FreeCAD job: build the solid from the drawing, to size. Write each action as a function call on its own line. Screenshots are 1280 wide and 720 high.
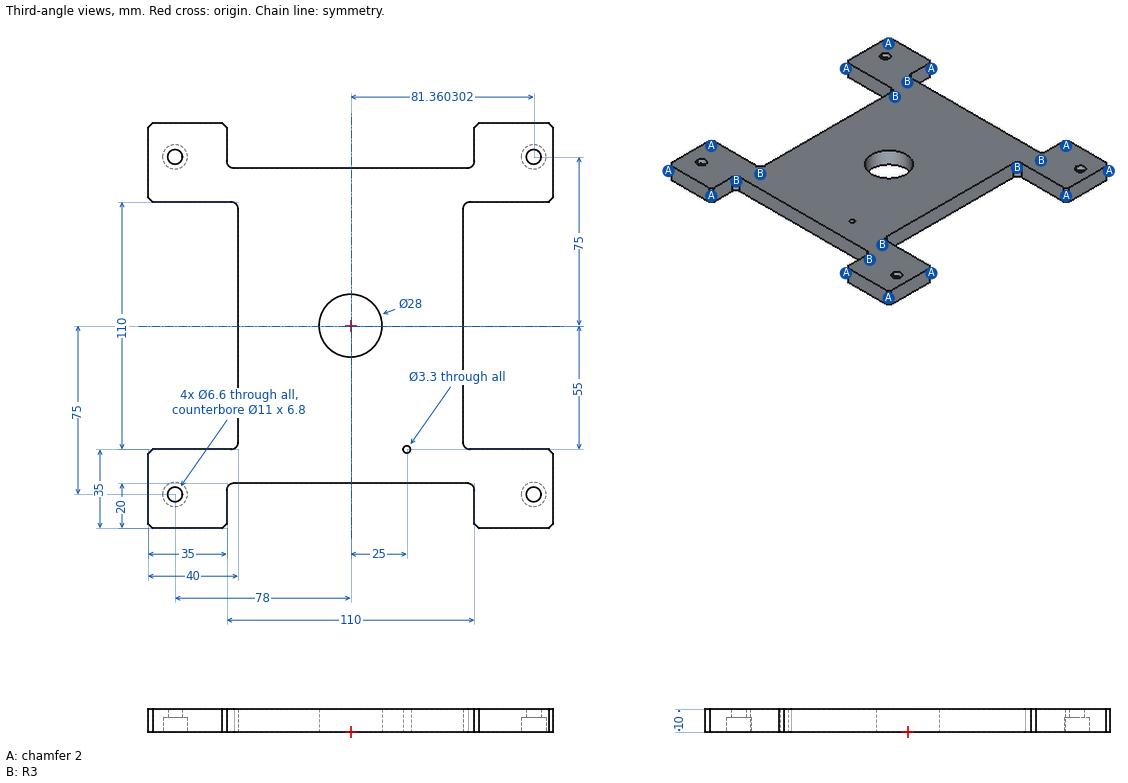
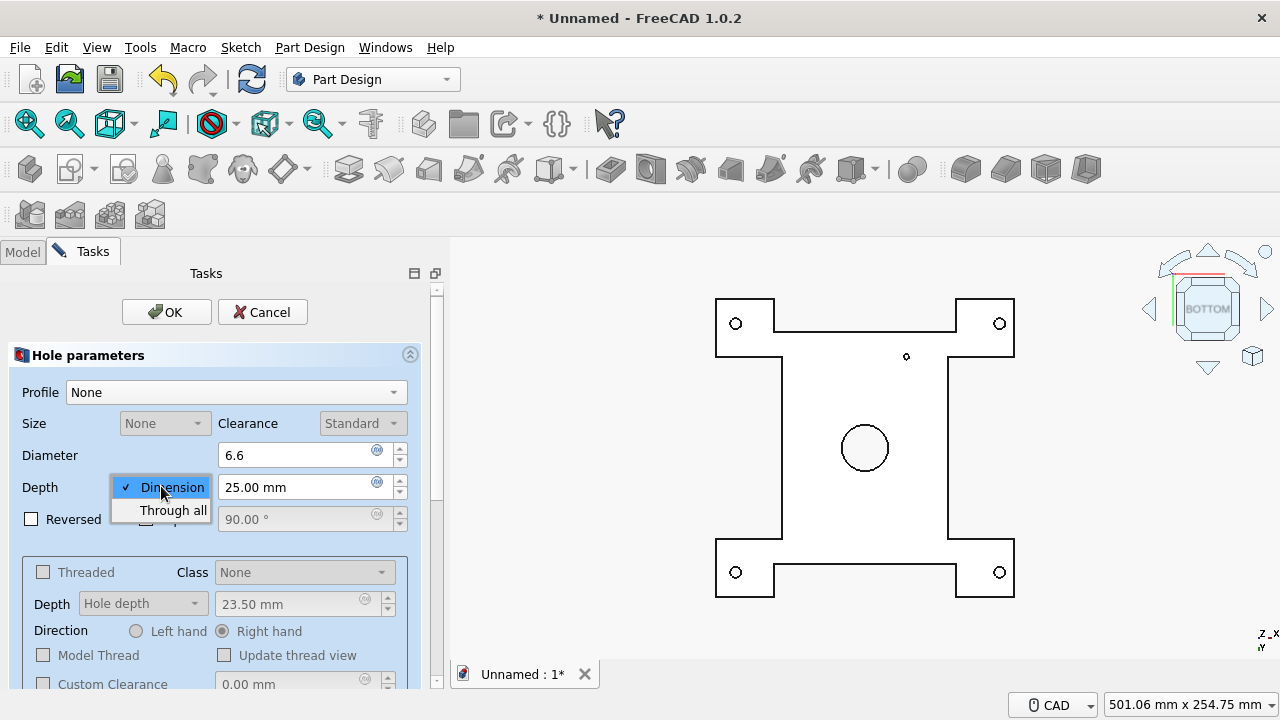
click(160, 510)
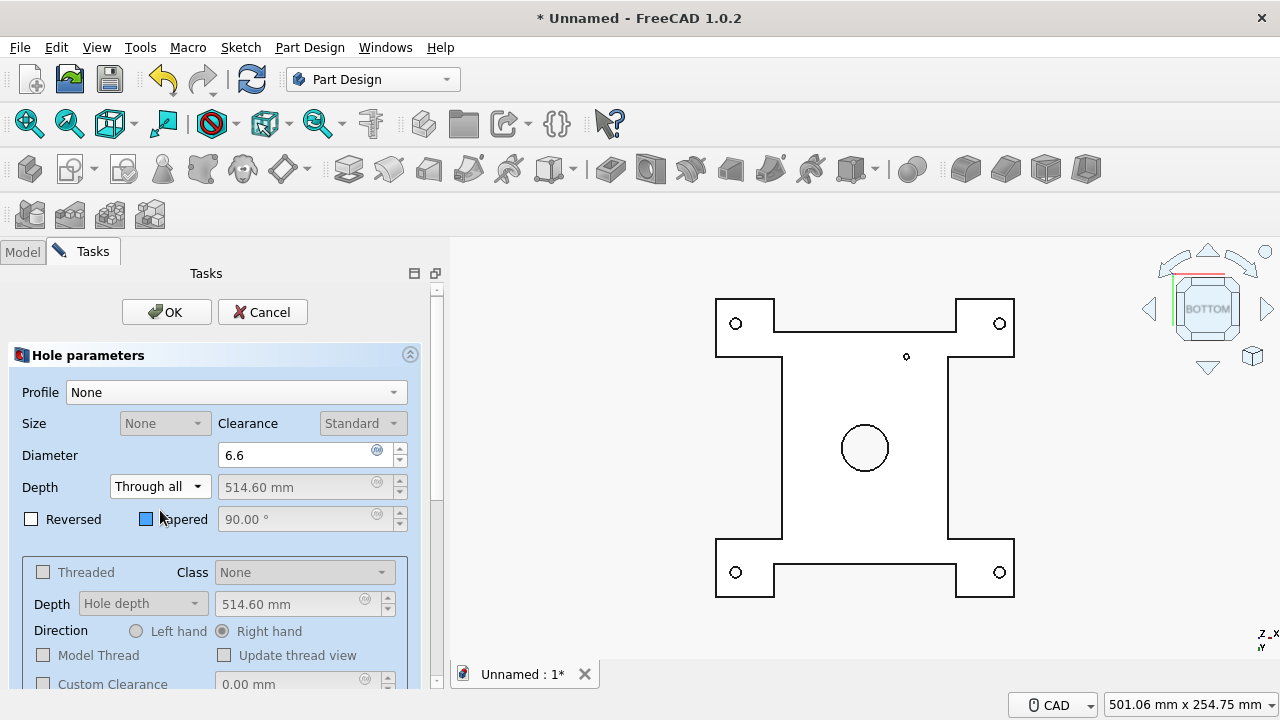
scroll(437, 486, down, 3)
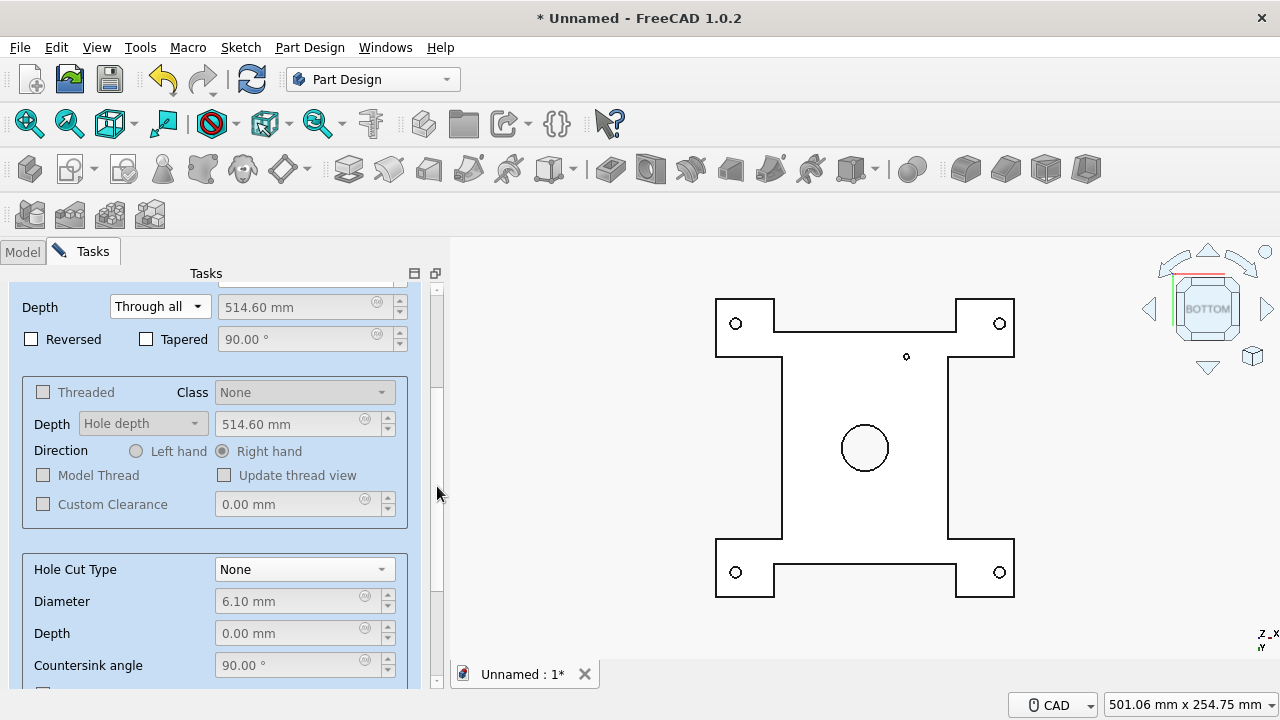
click(306, 570)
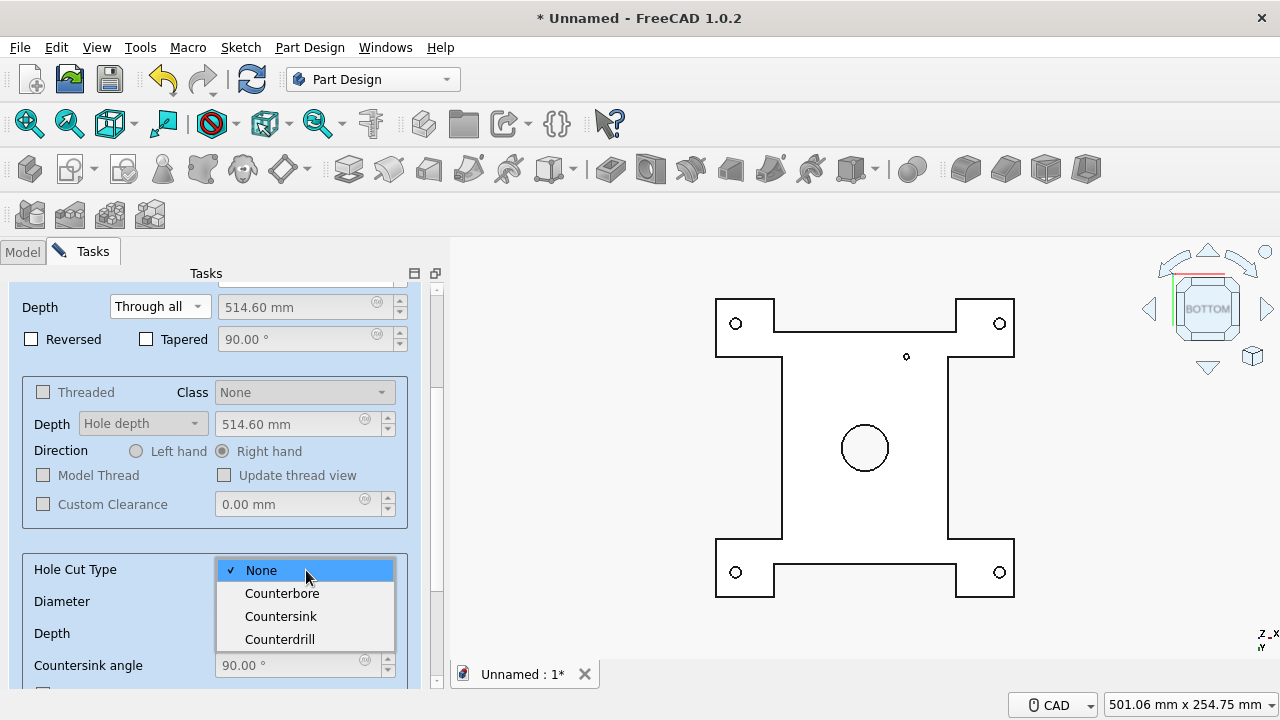
click(304, 594)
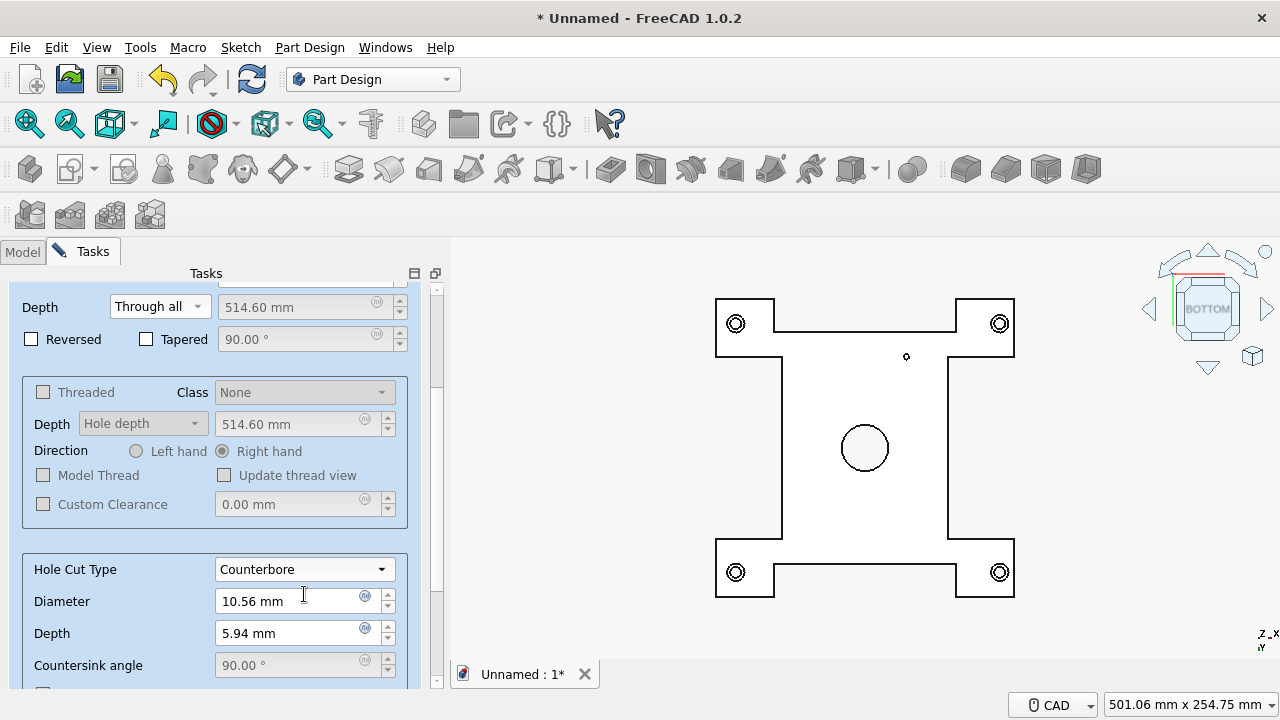
triple_click(298, 601)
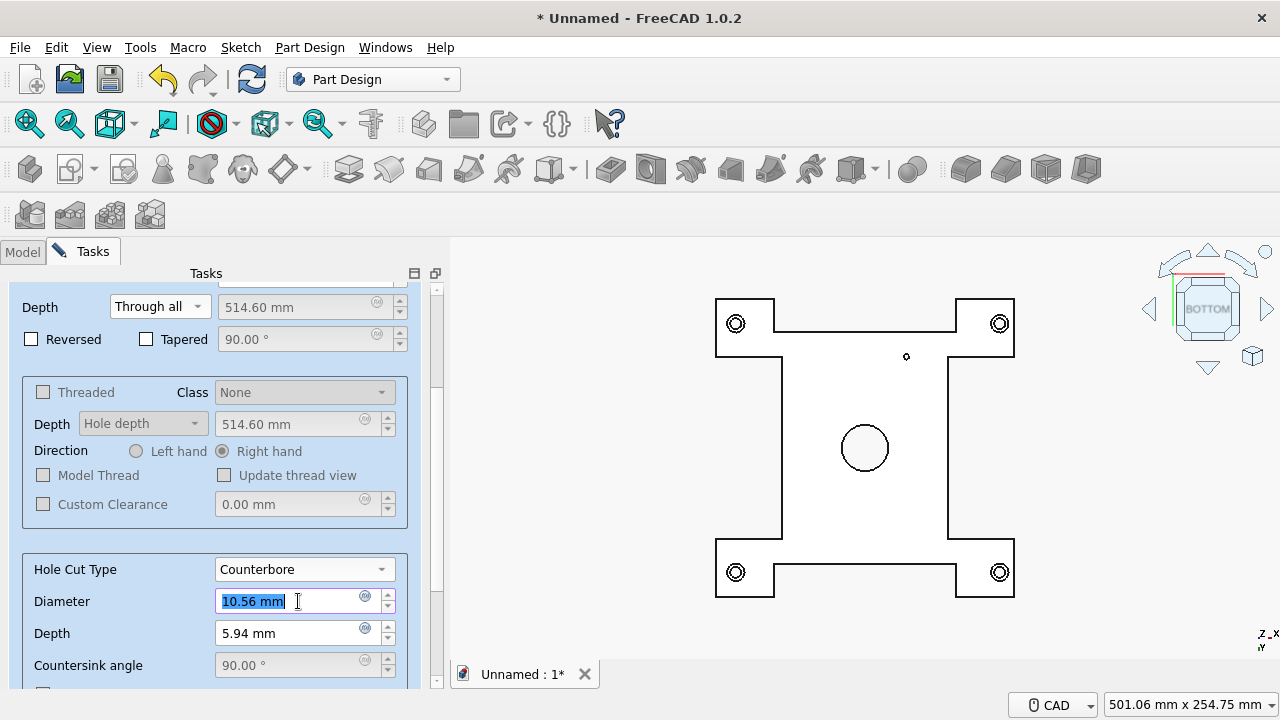
text(11)
key(Tab)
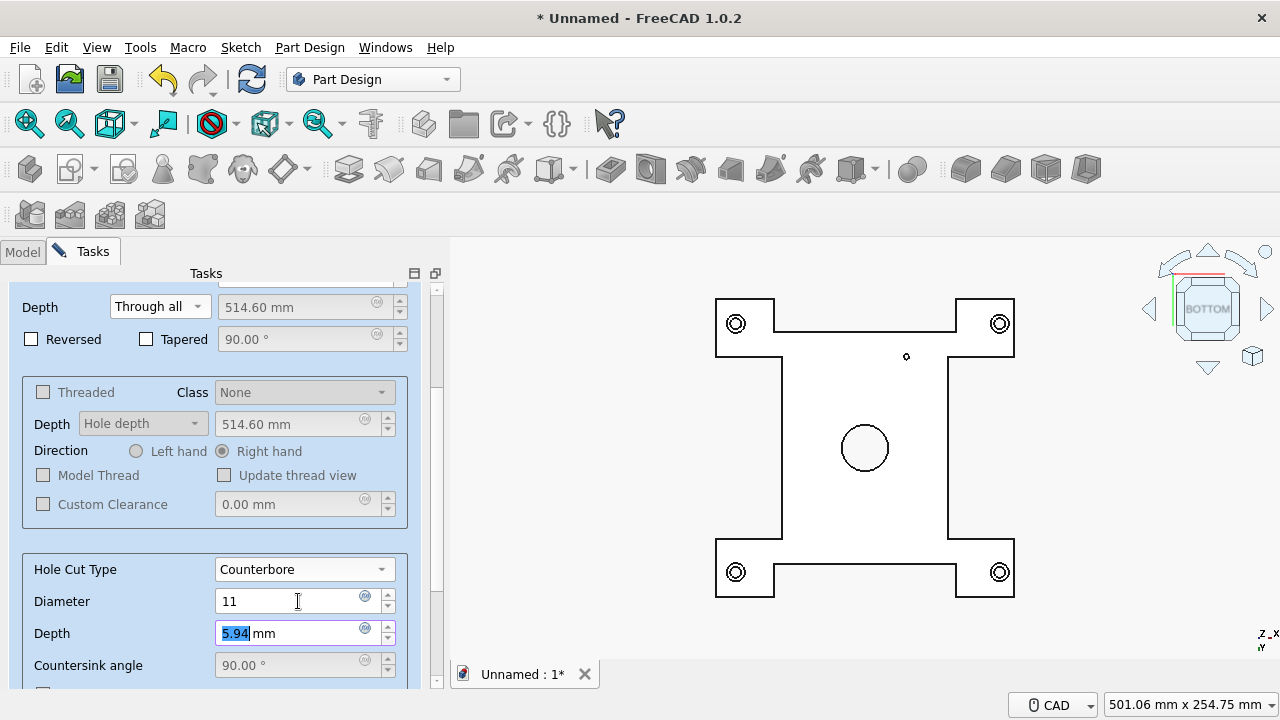
text(6.8)
key(Tab)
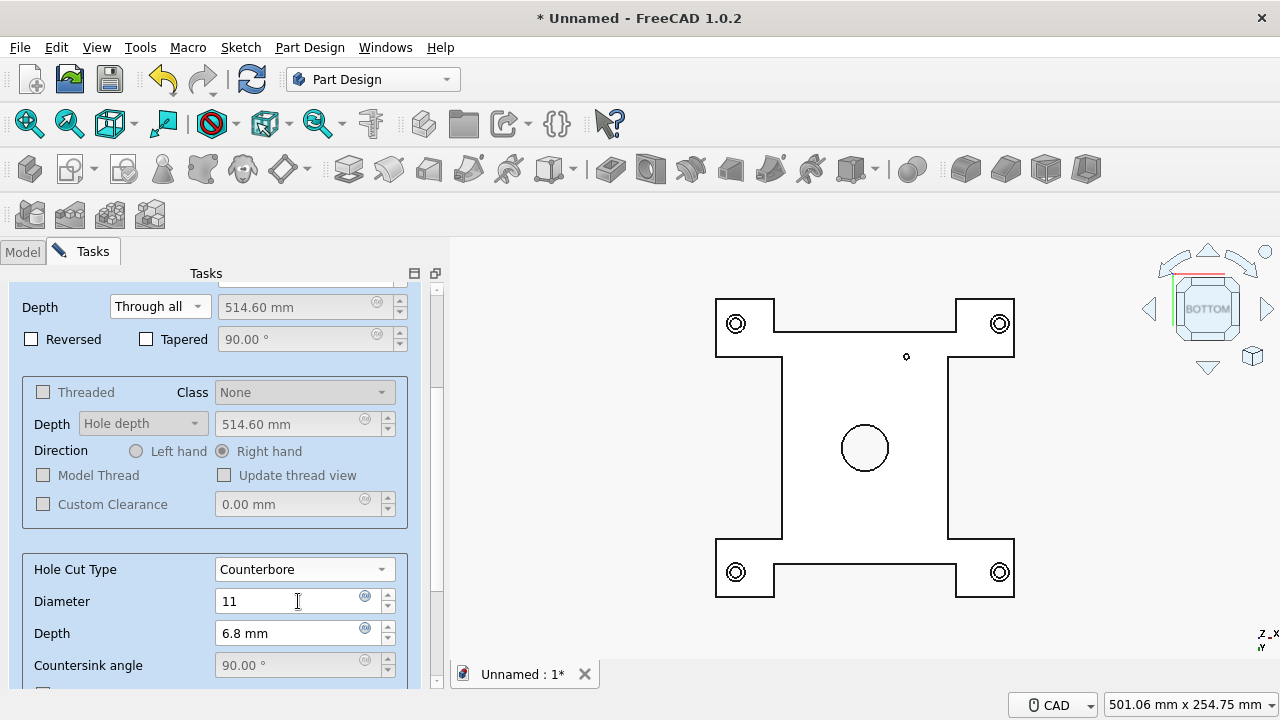
scroll(437, 486, up, 4)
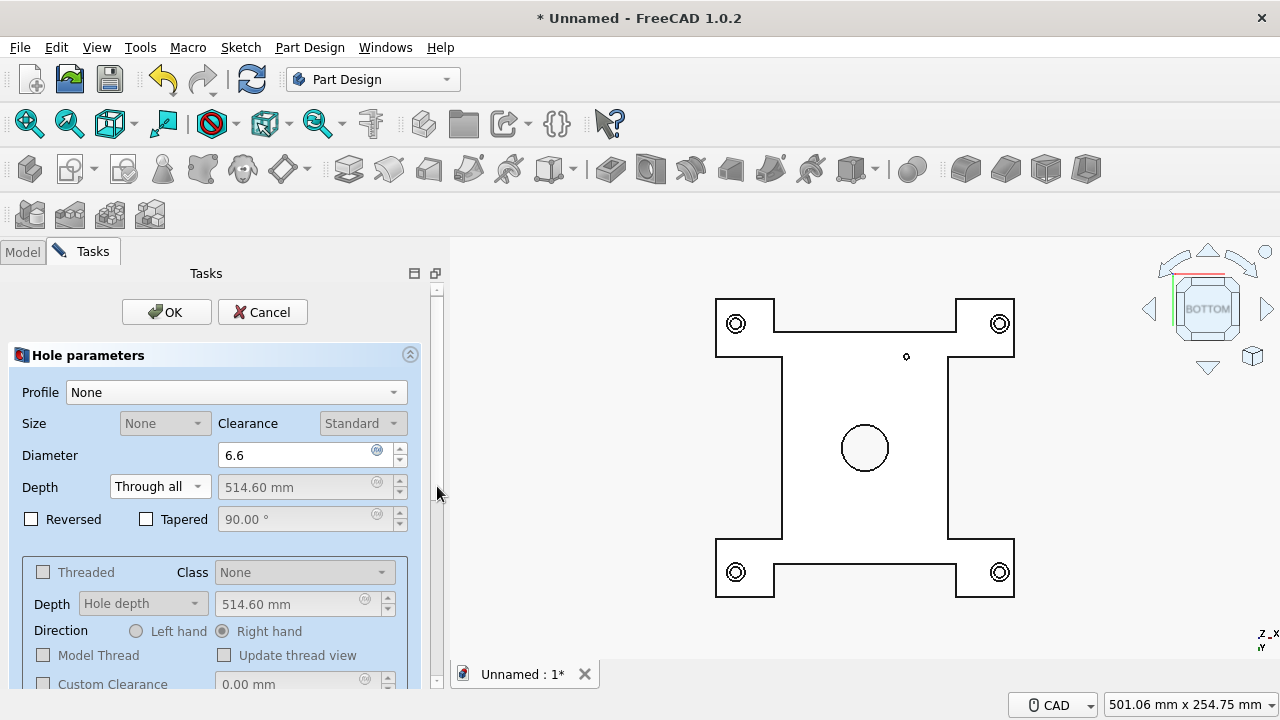
click(167, 312)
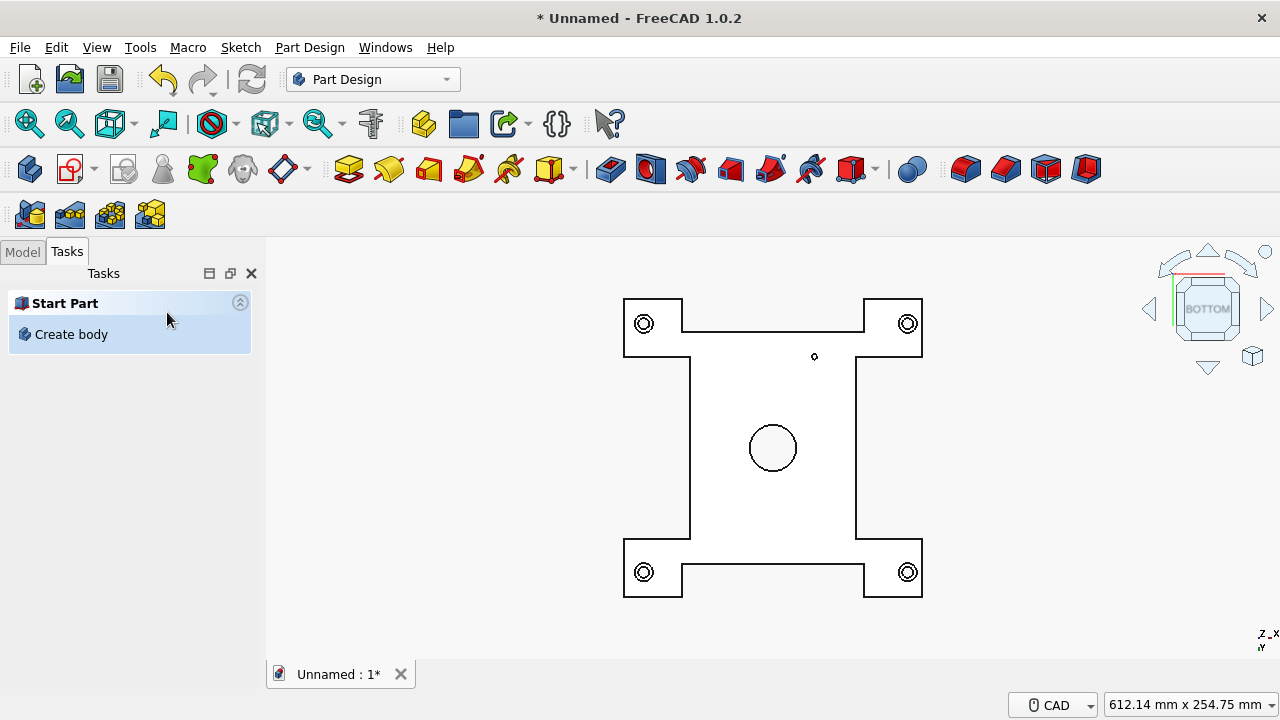
scroll(624, 538, up, 5)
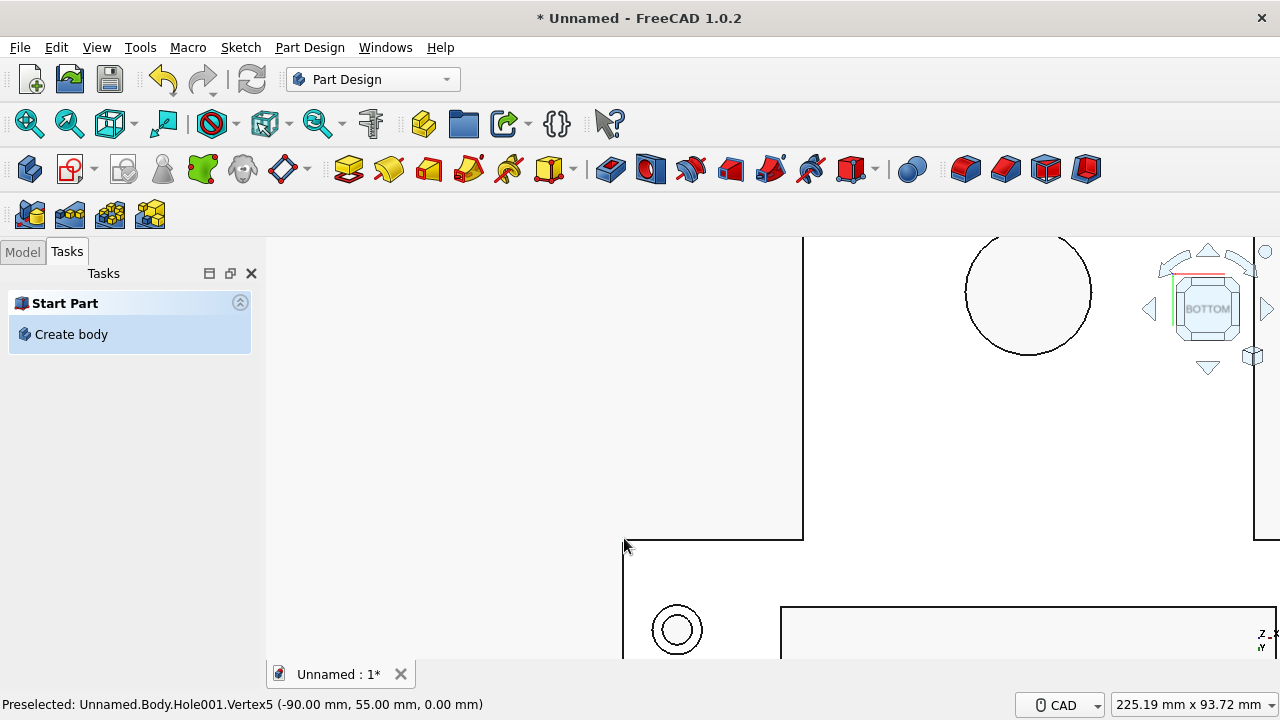
click(30, 124)